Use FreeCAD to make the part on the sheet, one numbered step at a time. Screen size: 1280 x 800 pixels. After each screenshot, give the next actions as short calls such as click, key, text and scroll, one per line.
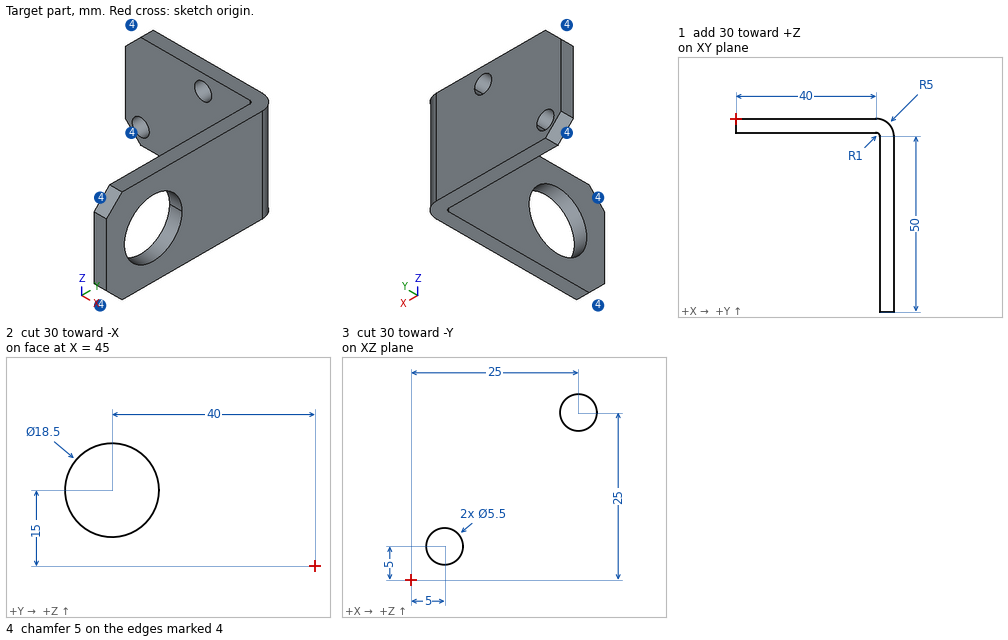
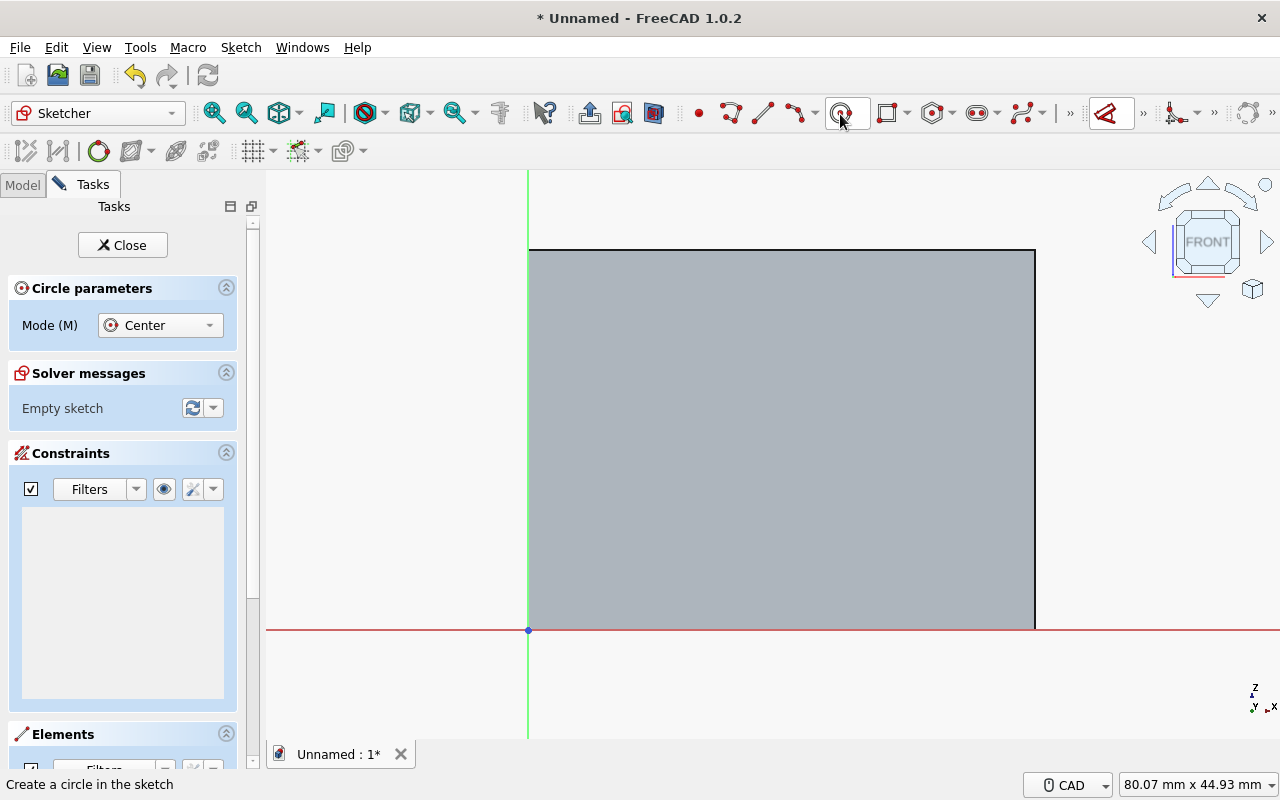
click(592, 567)
click(616, 542)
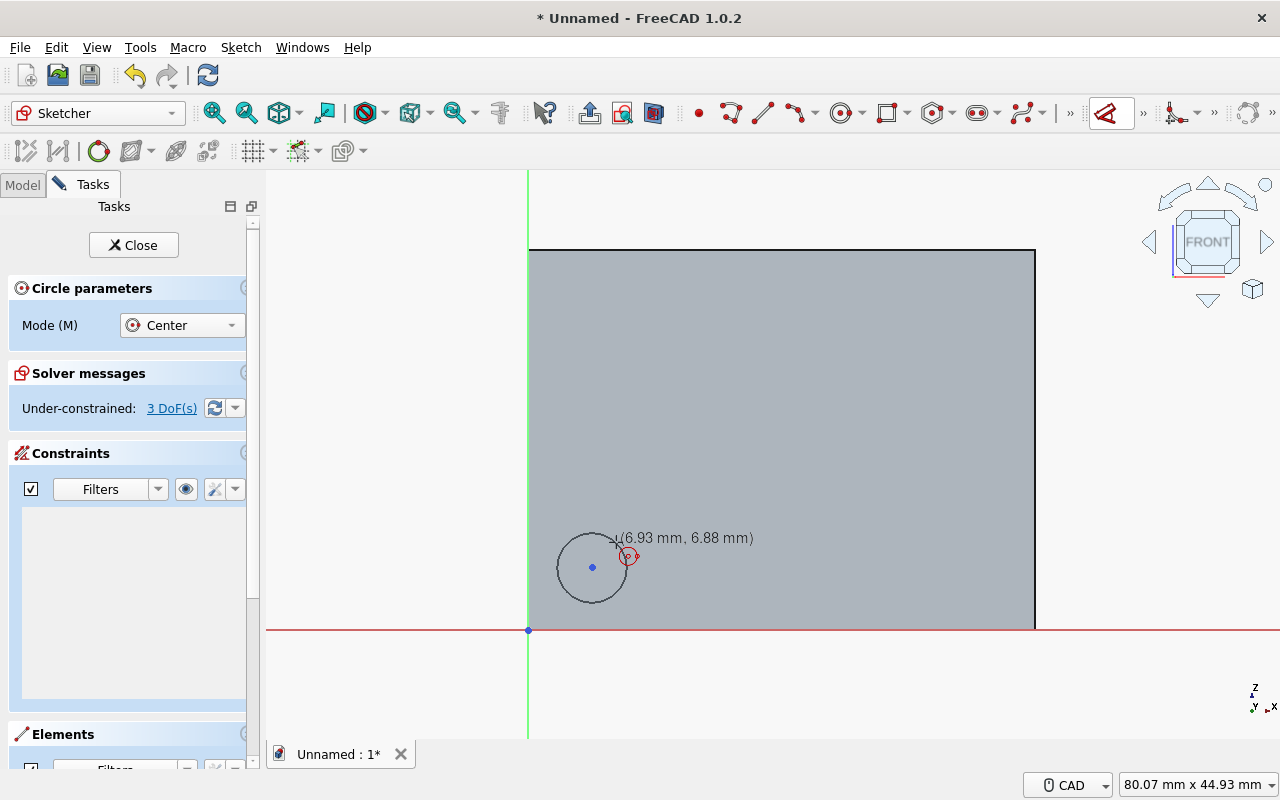
click(845, 313)
click(869, 289)
key(Escape)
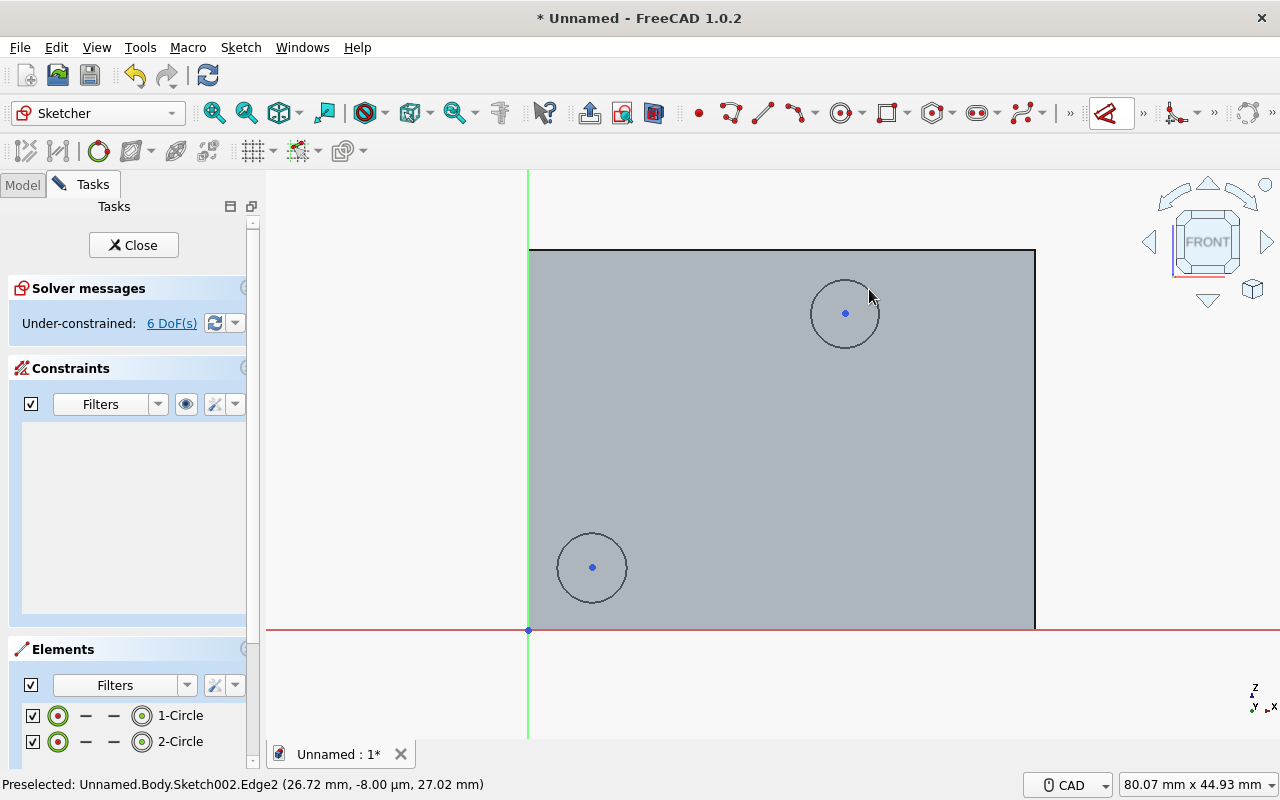
click(616, 543)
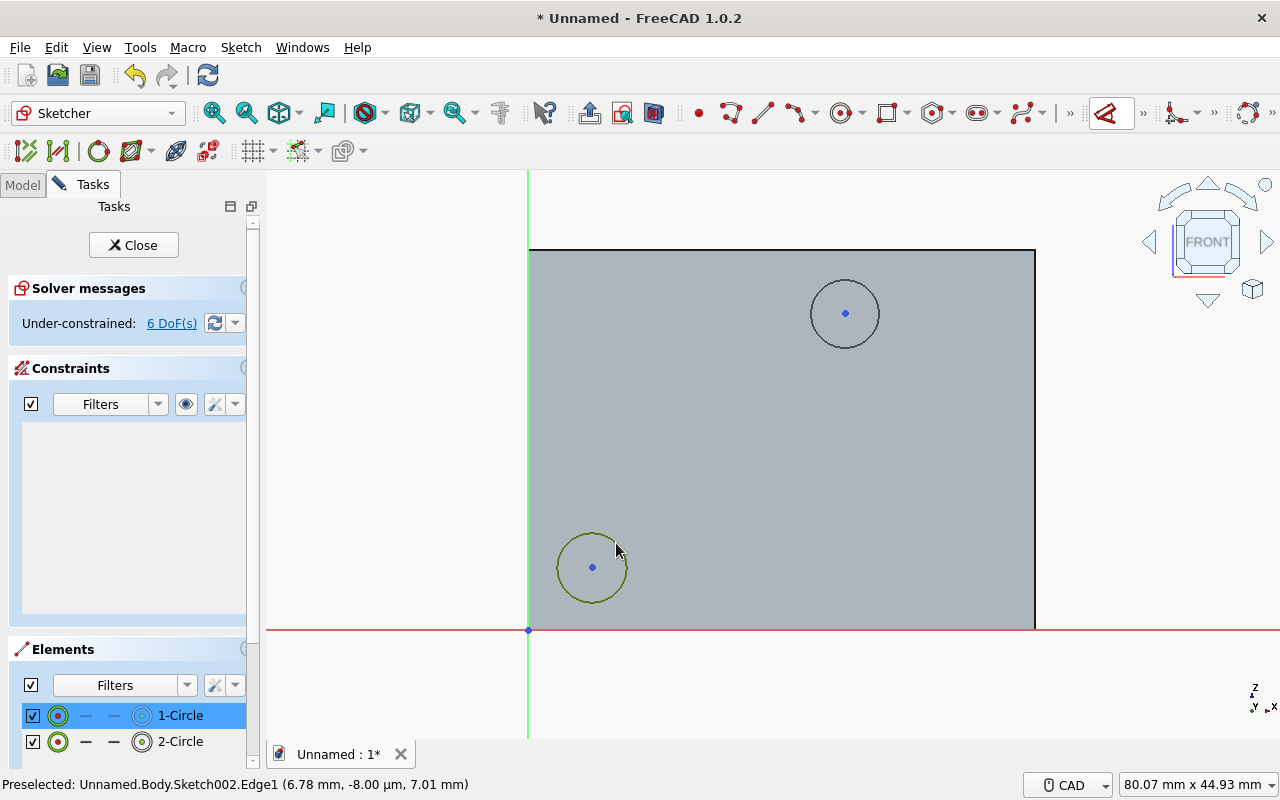
click(869, 290)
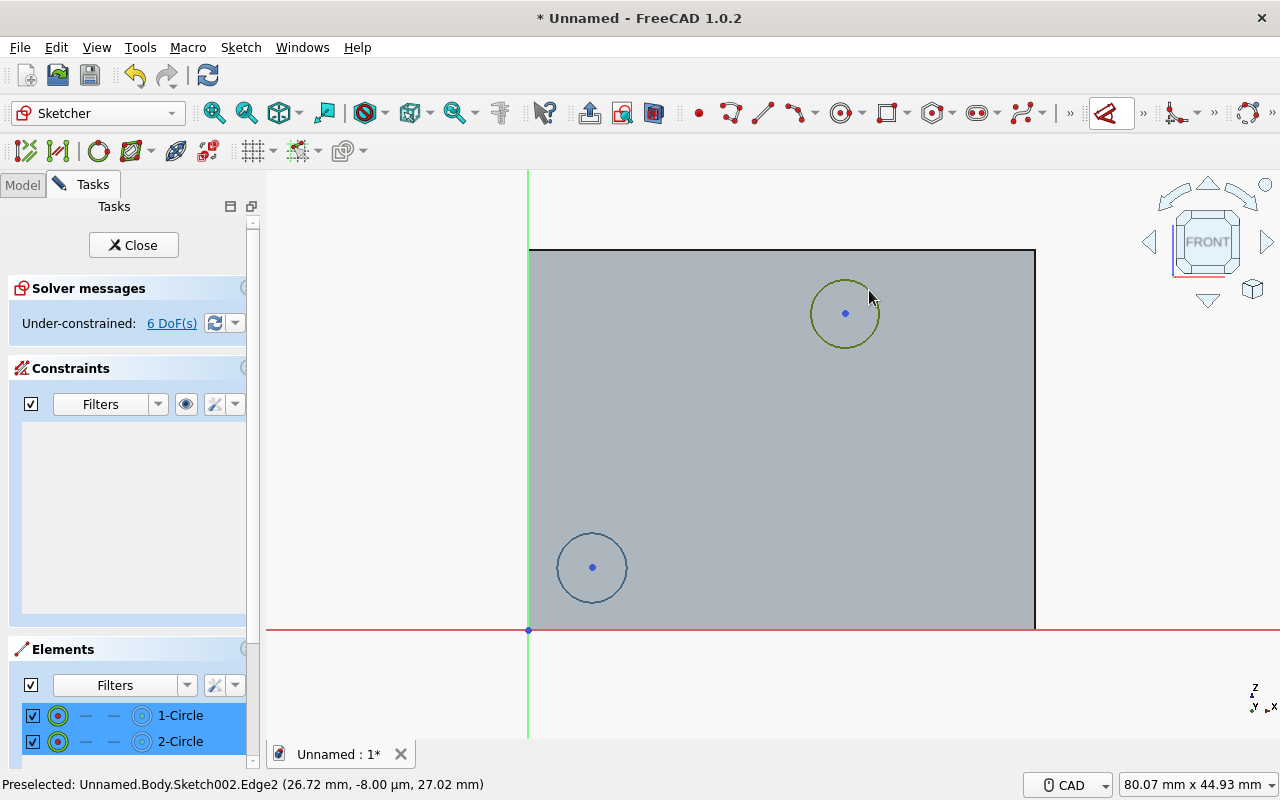
key(e)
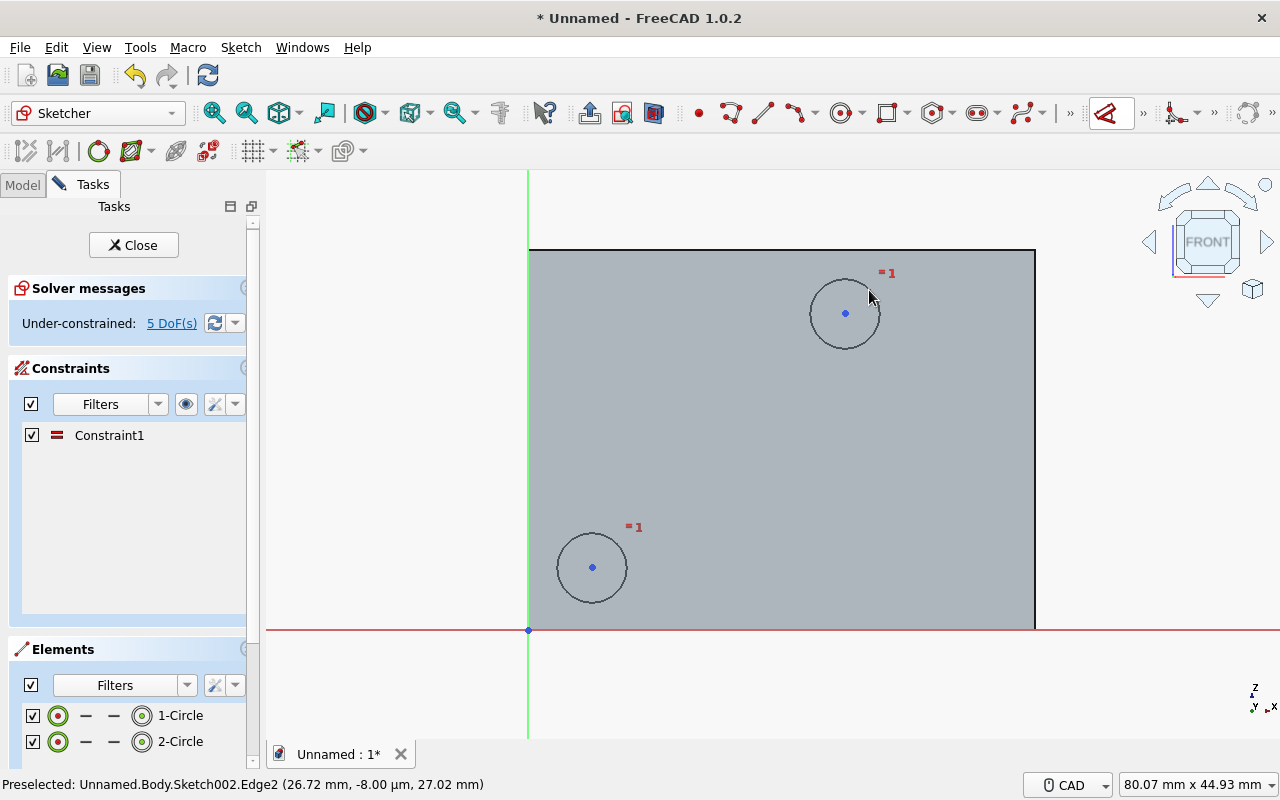
click(616, 543)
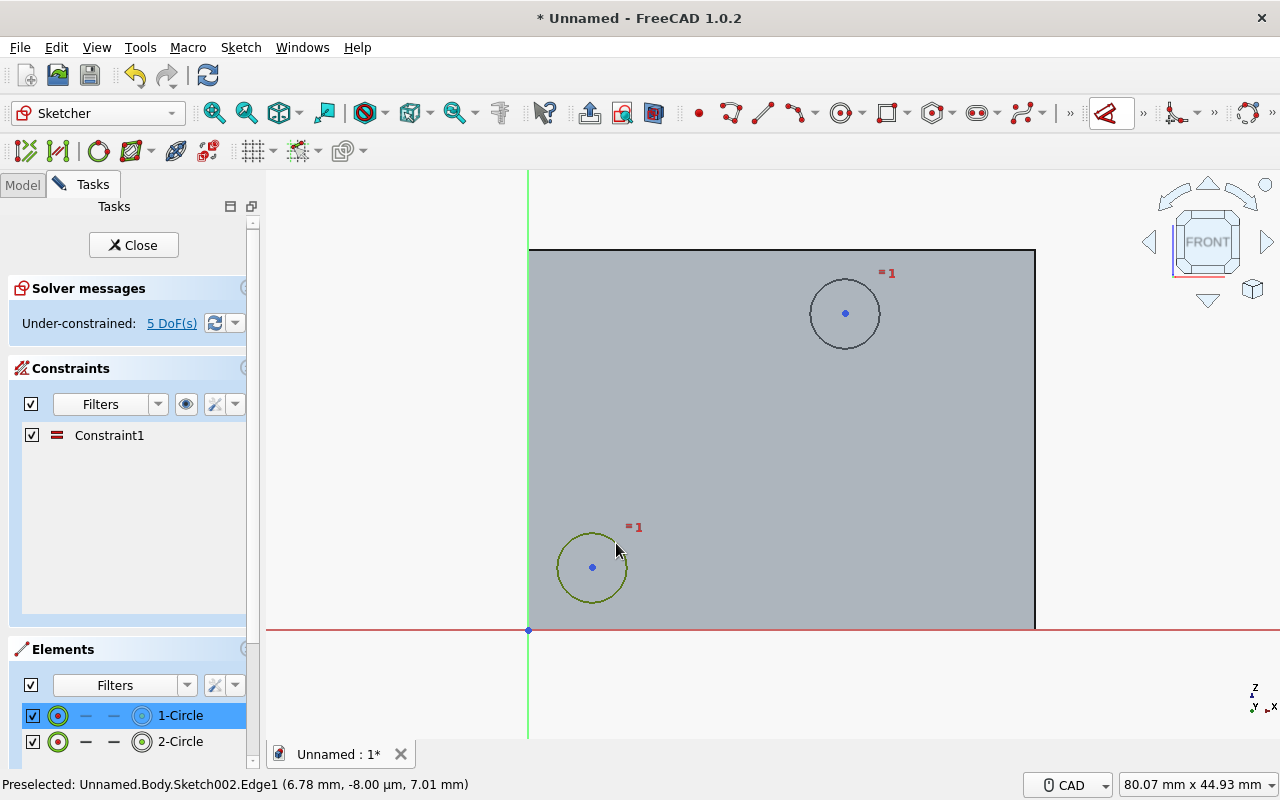
key(k)
key(o)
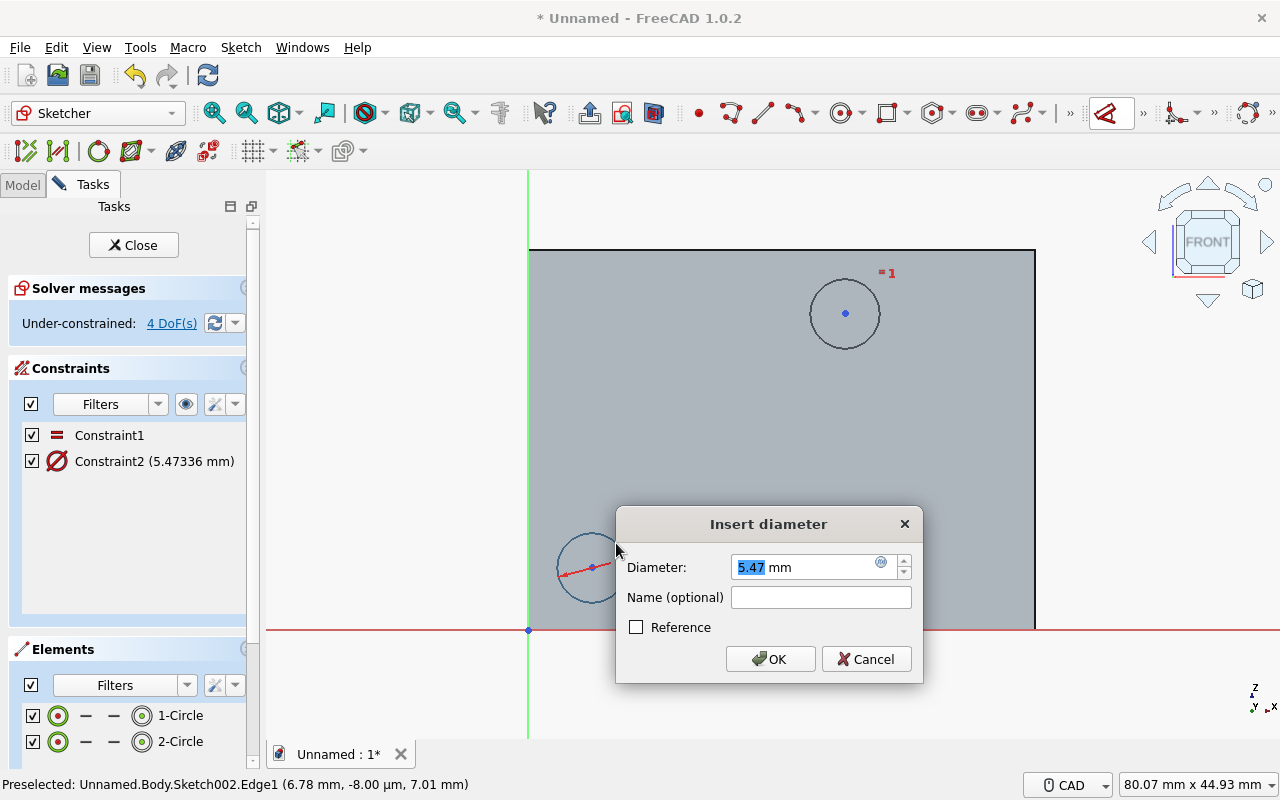
text(5.5)
key(Return)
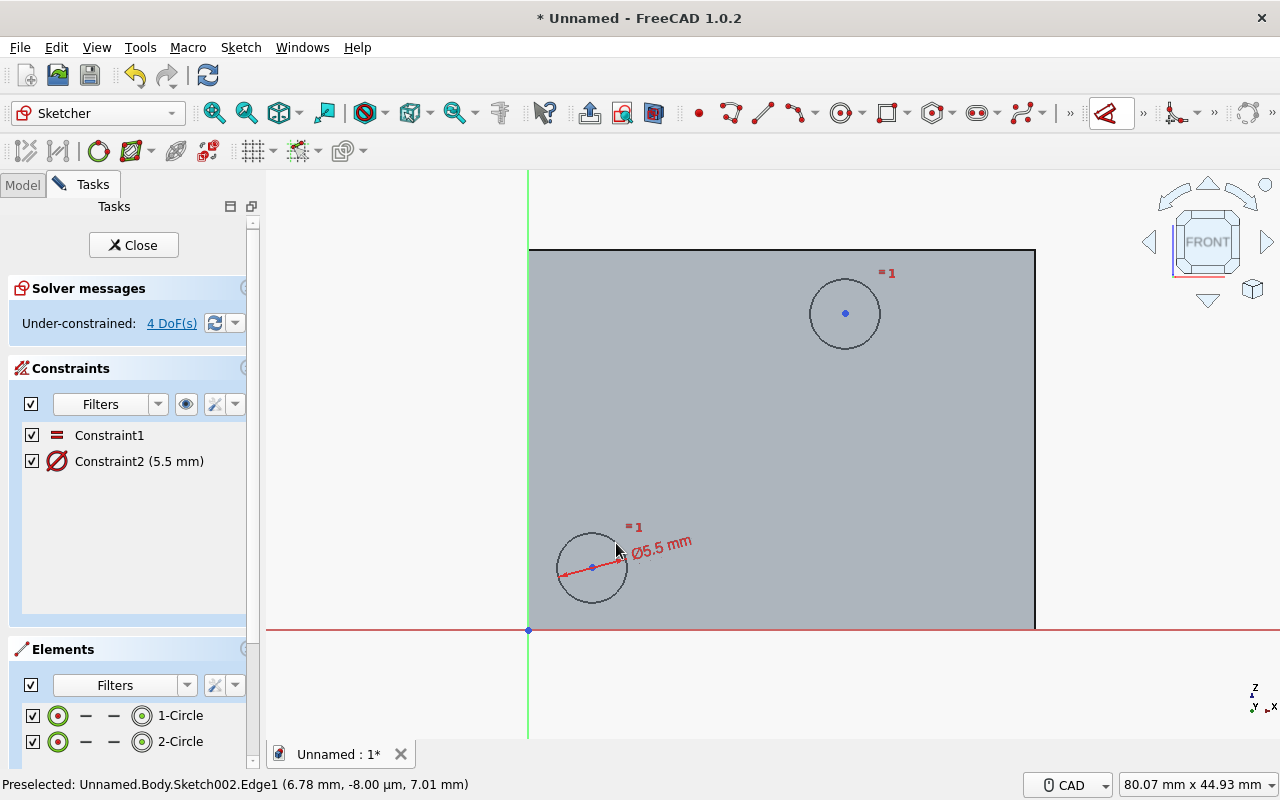
click(592, 568)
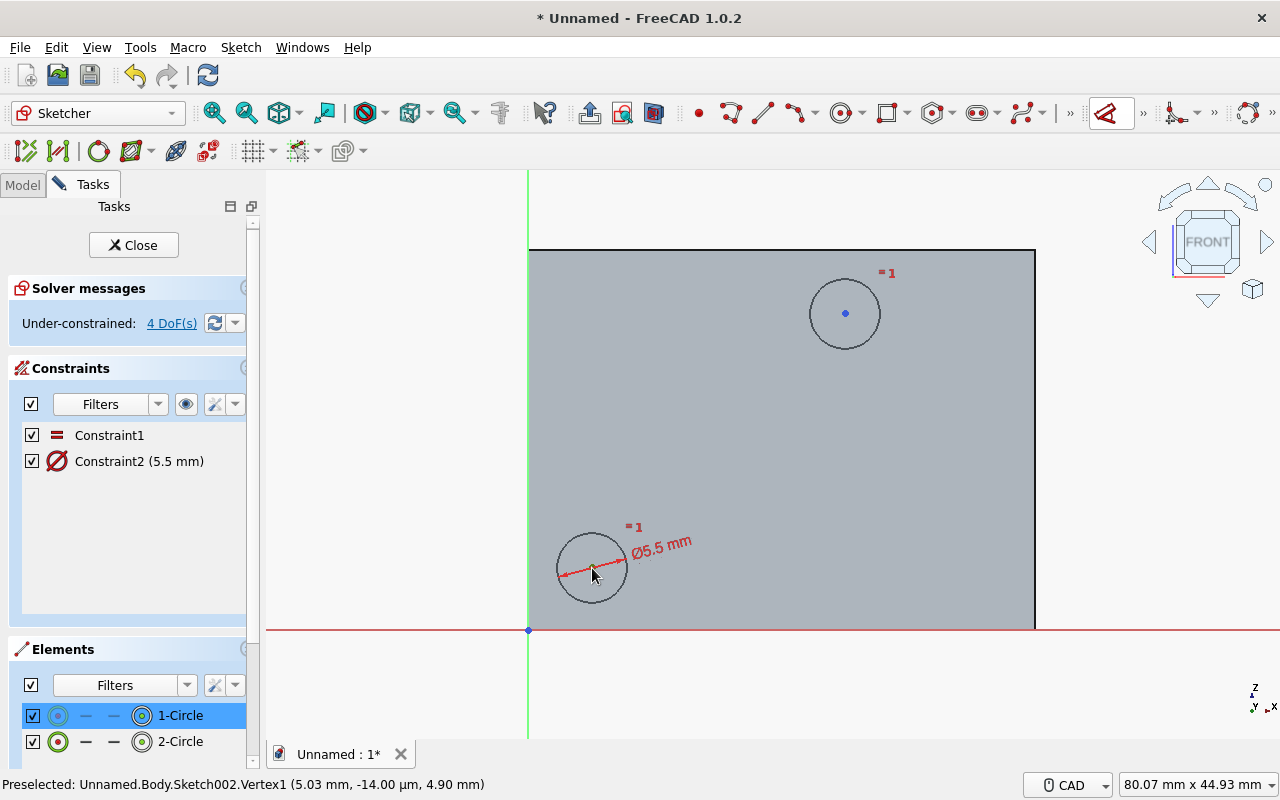
click(1128, 114)